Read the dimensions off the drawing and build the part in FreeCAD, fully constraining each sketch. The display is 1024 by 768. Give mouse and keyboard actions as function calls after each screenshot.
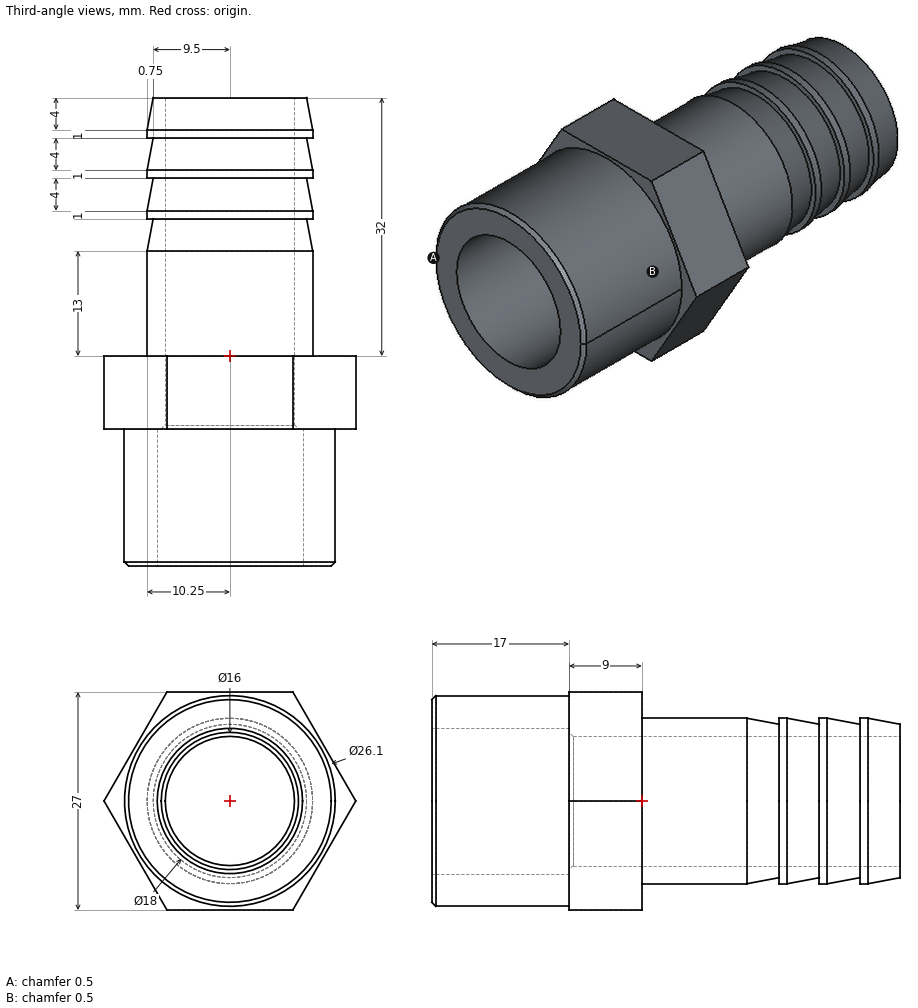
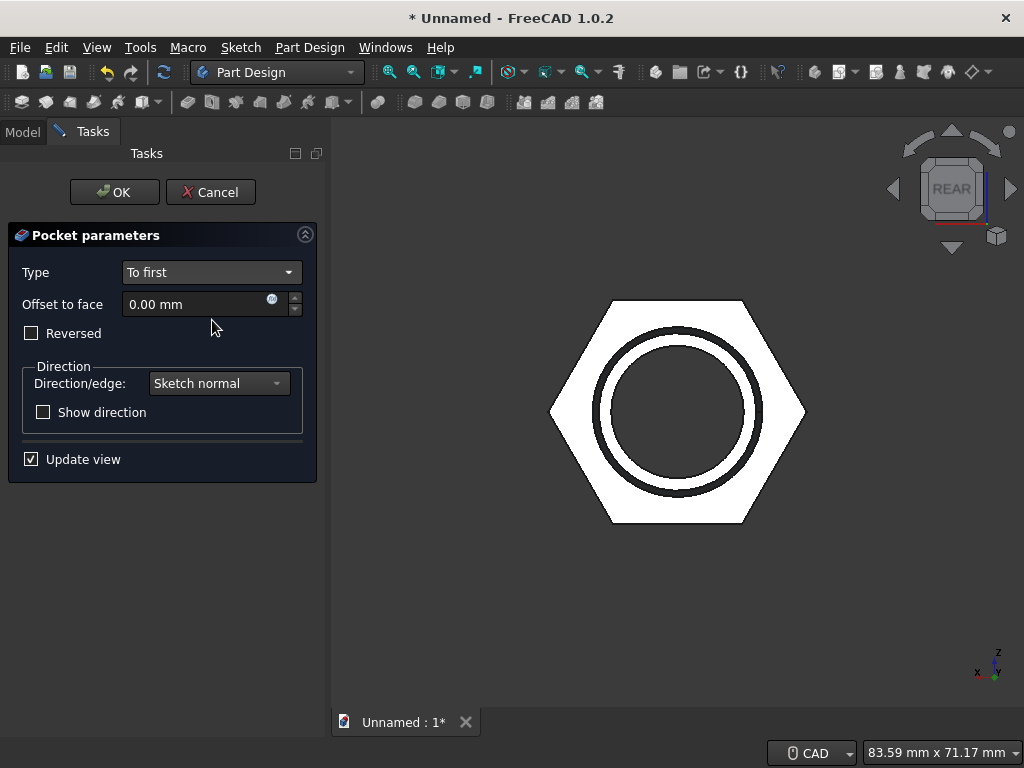
click(115, 192)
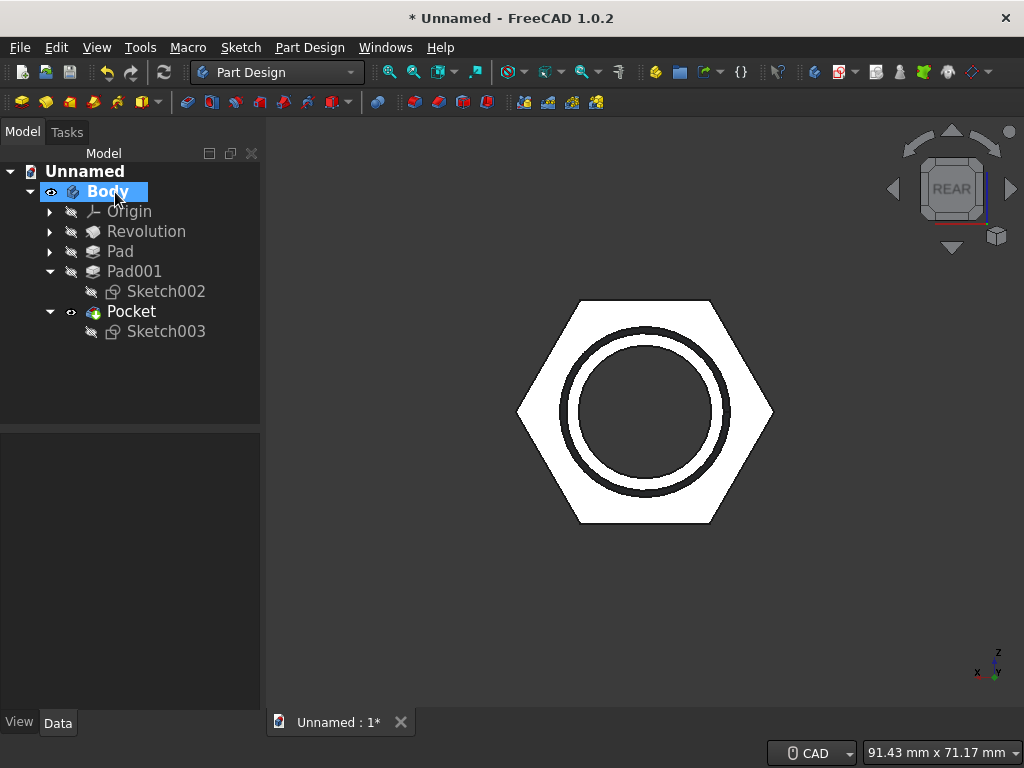
key(v)
key(f)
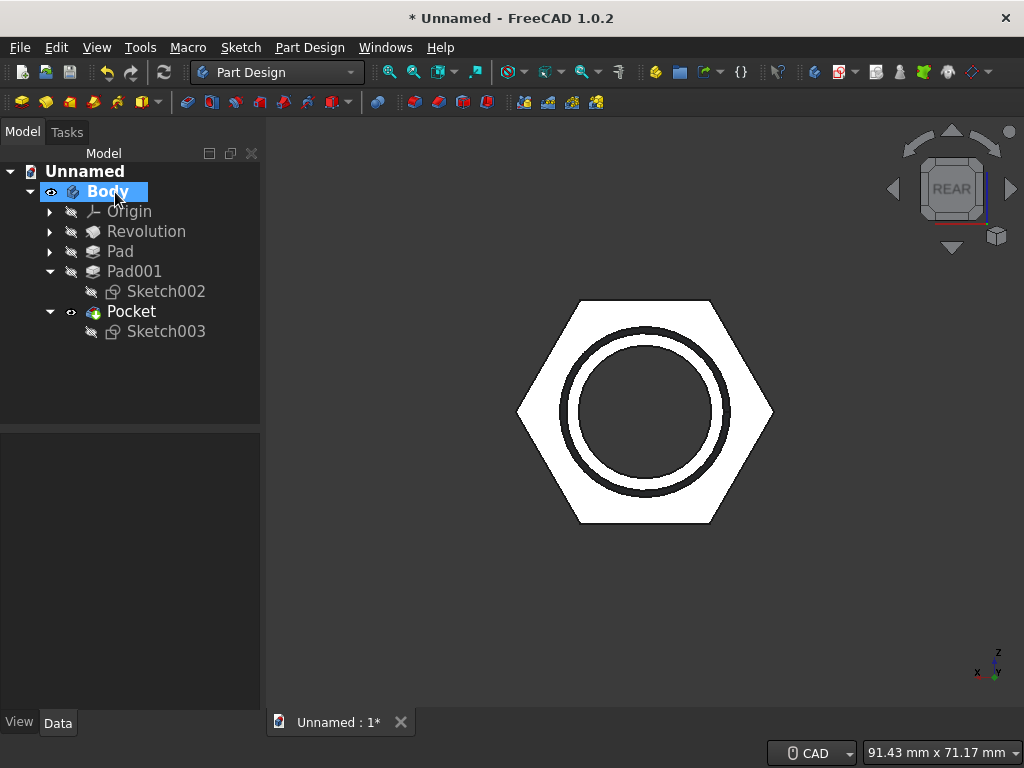
key(0)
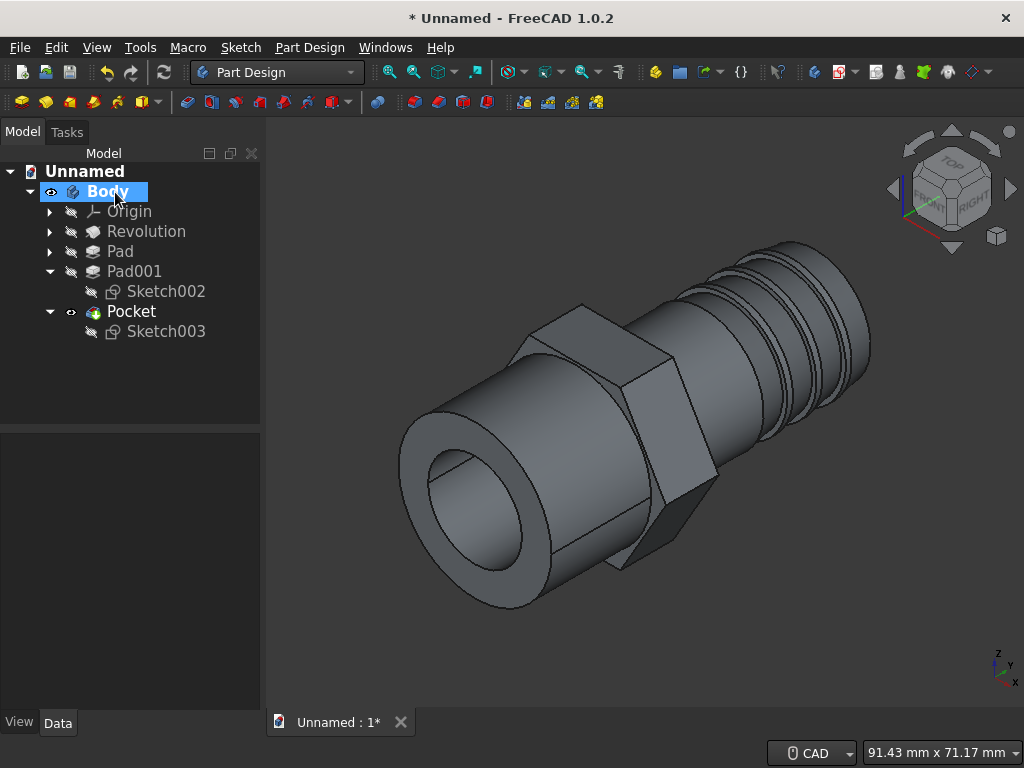
click(431, 534)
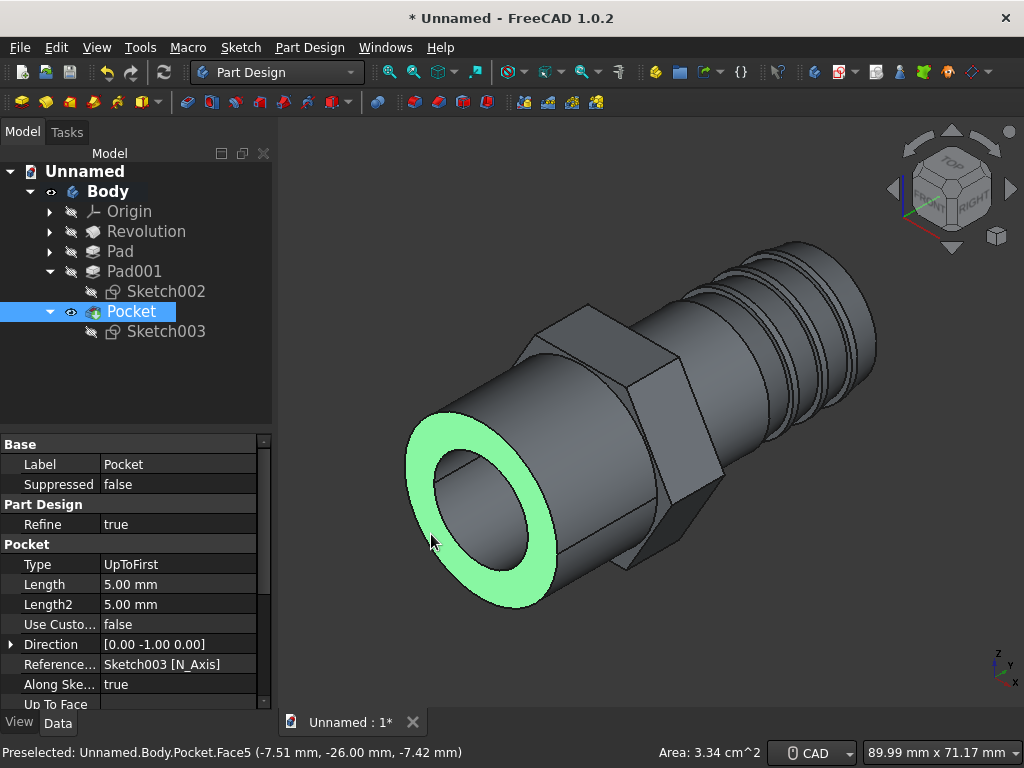
click(840, 72)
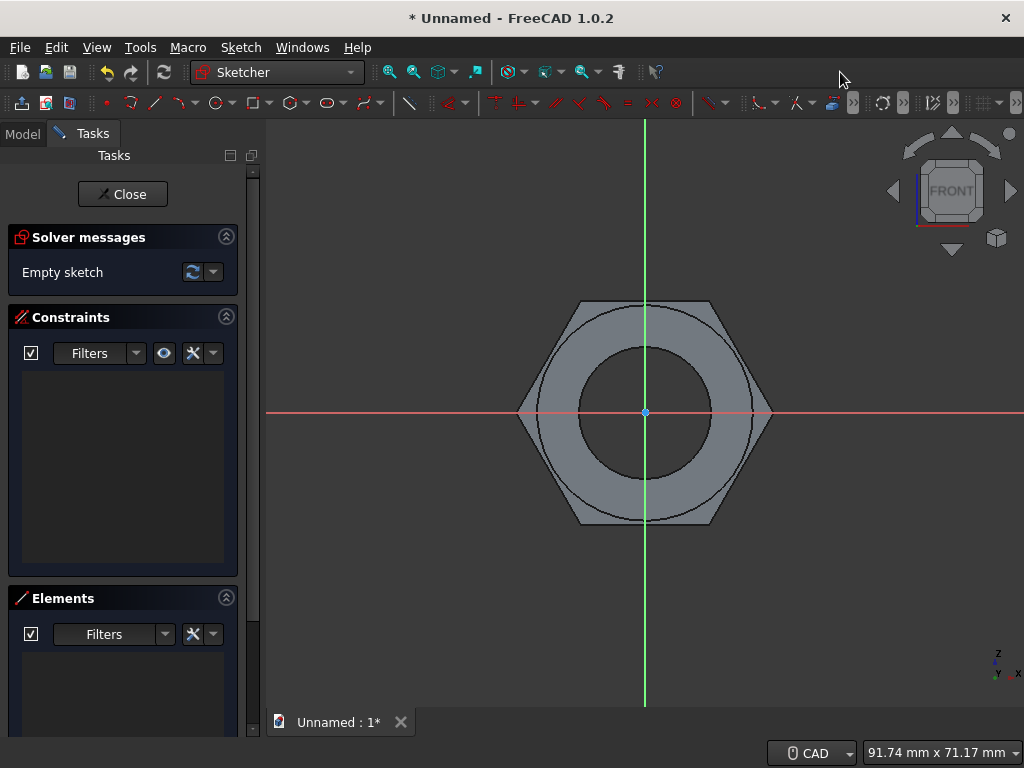
scroll(685, 413, up, 5)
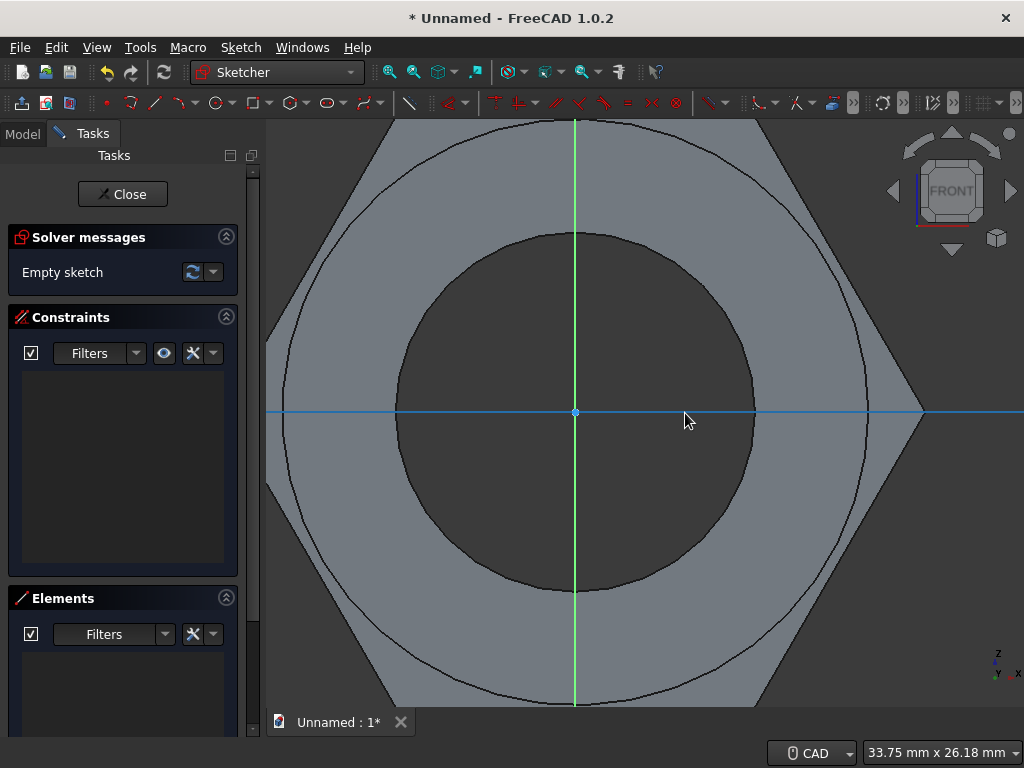
key(g)
key(c)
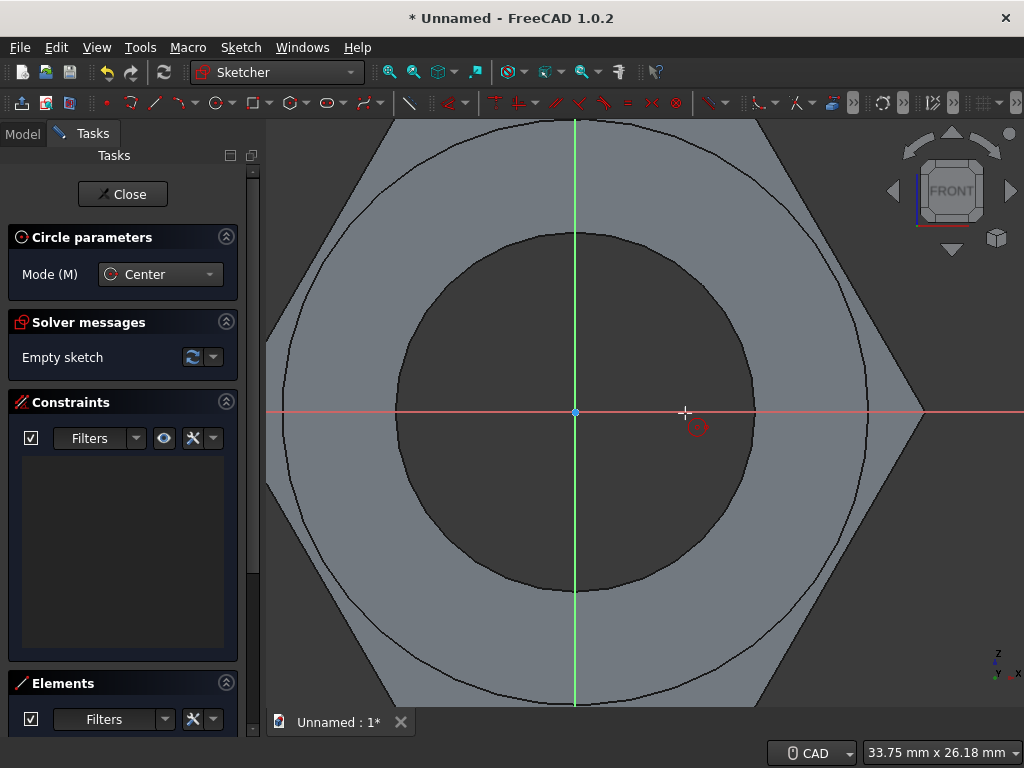
click(575, 412)
click(718, 269)
key(Escape)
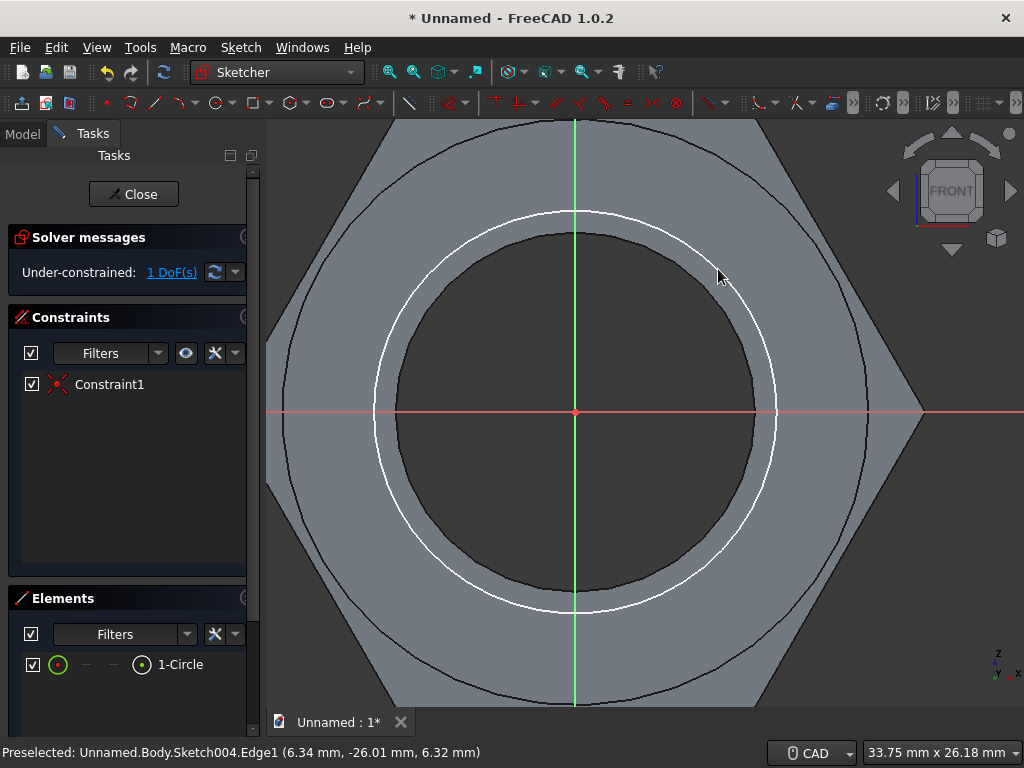
click(448, 104)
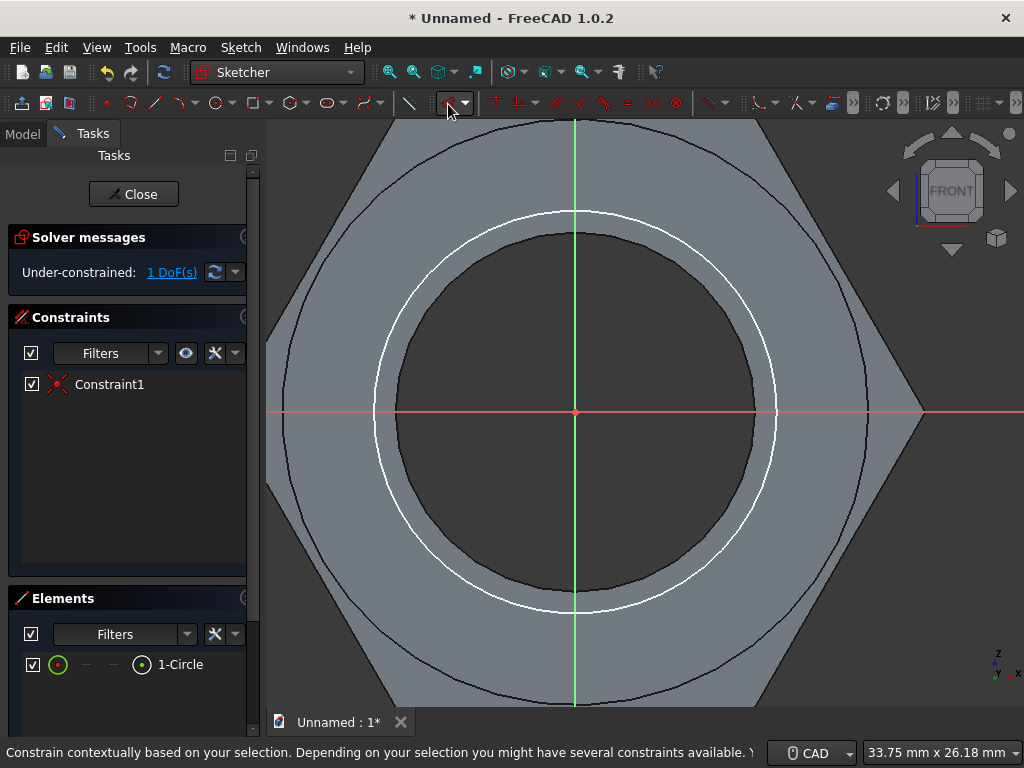
click(717, 269)
click(740, 246)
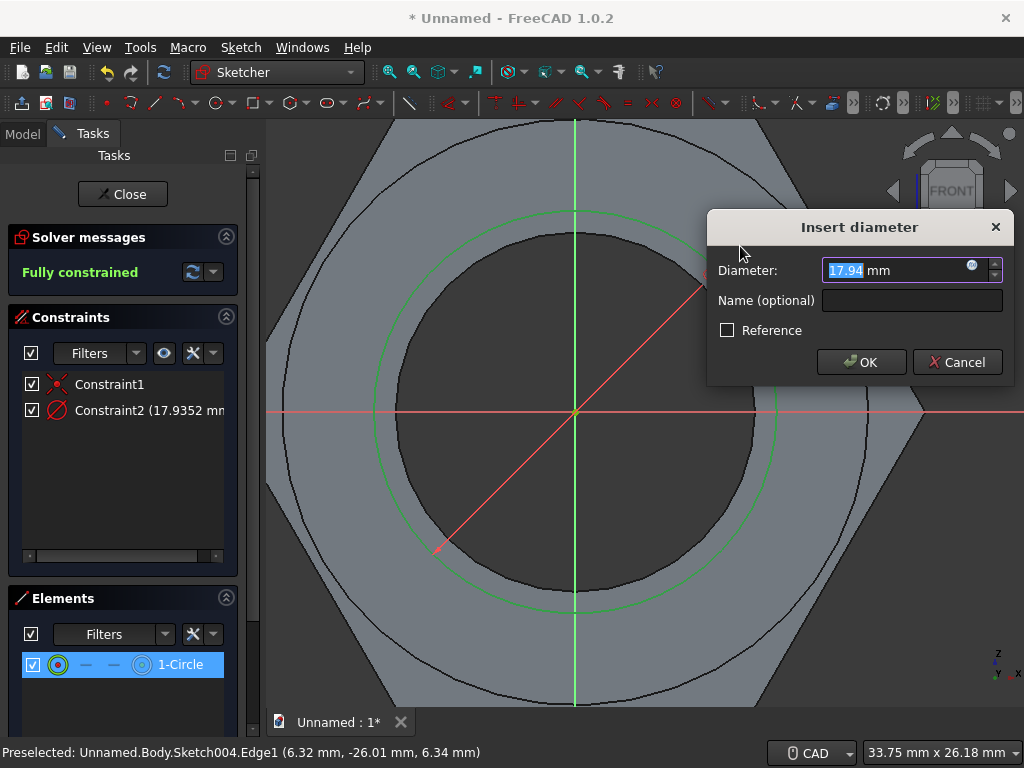
text(18)
key(Return)
key(Escape)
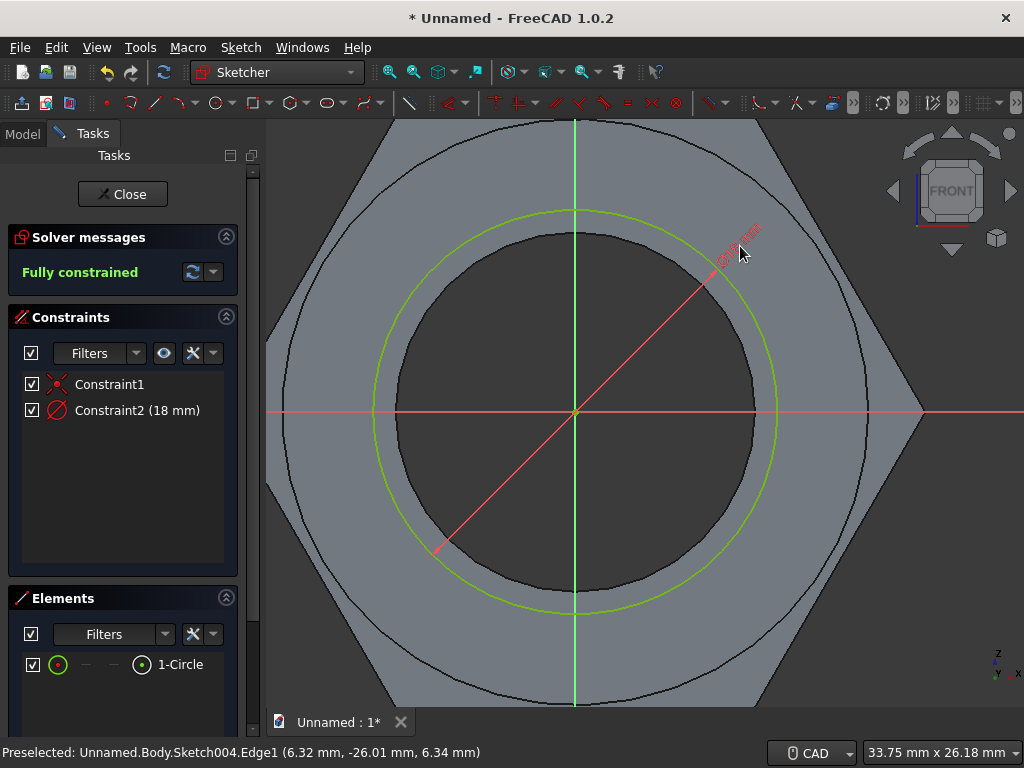
click(123, 194)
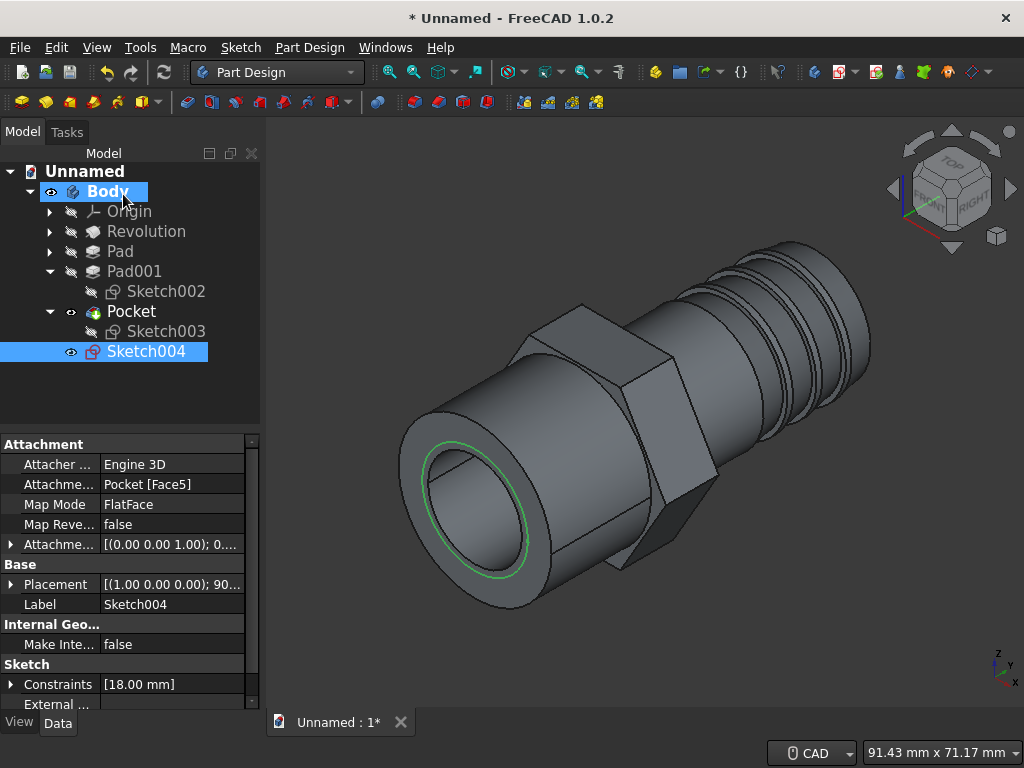
click(188, 102)